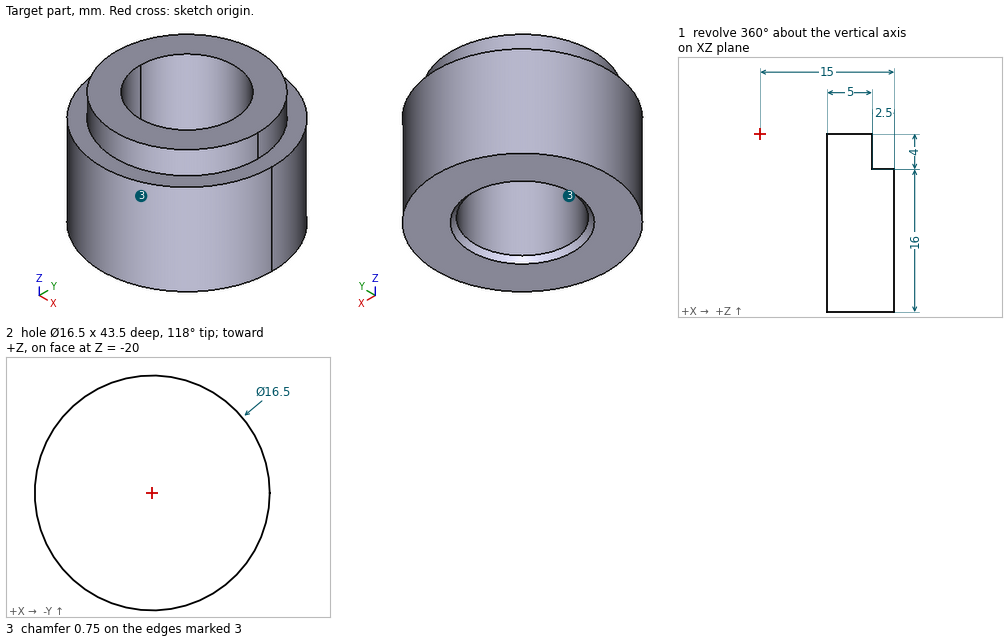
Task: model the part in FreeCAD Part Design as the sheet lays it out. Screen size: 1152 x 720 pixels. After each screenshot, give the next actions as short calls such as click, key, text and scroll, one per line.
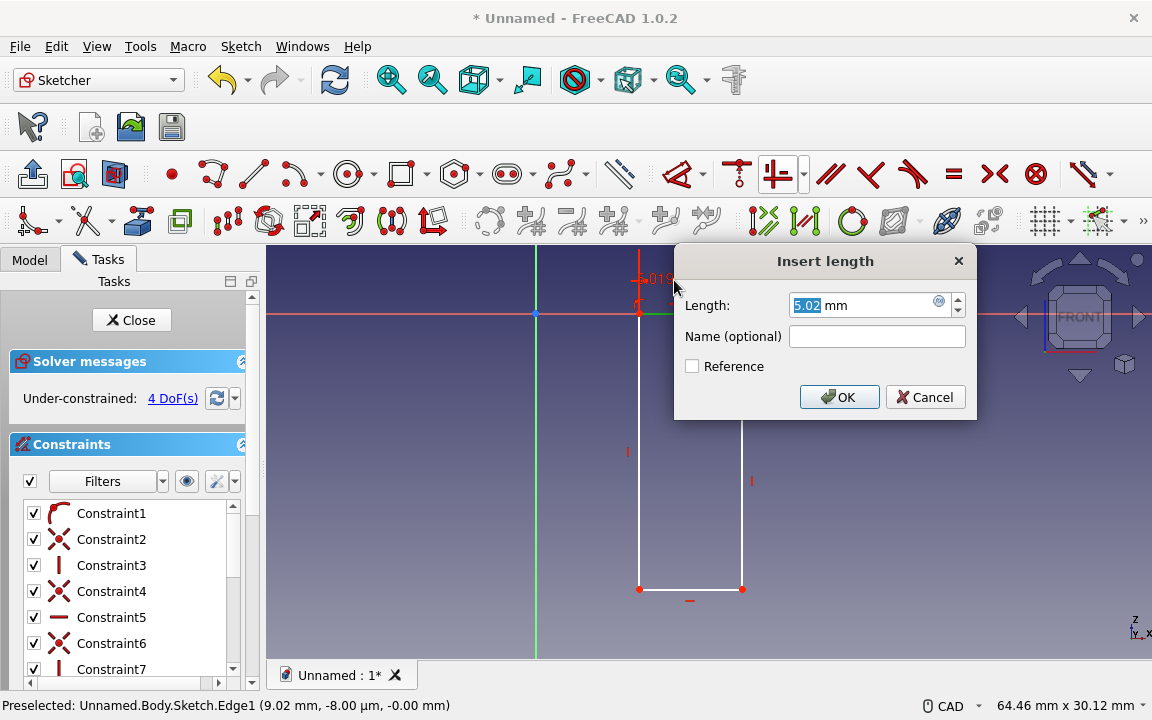
text(5)
key(Return)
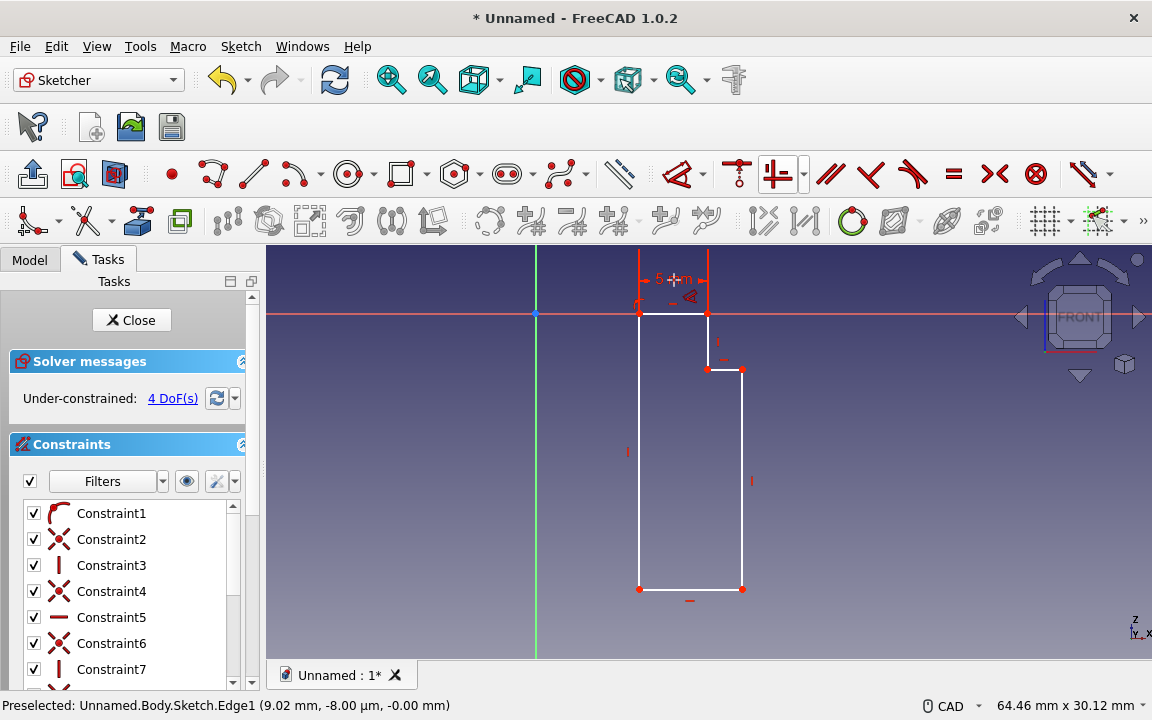
click(708, 331)
click(742, 342)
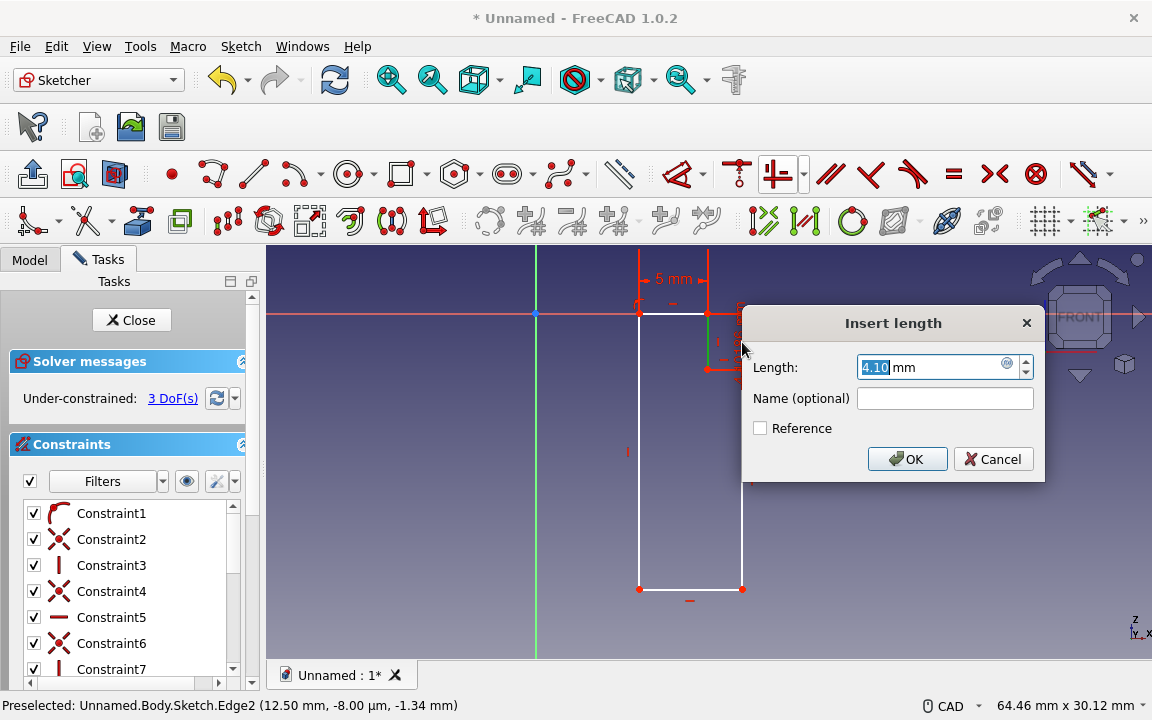
text(4)
key(Return)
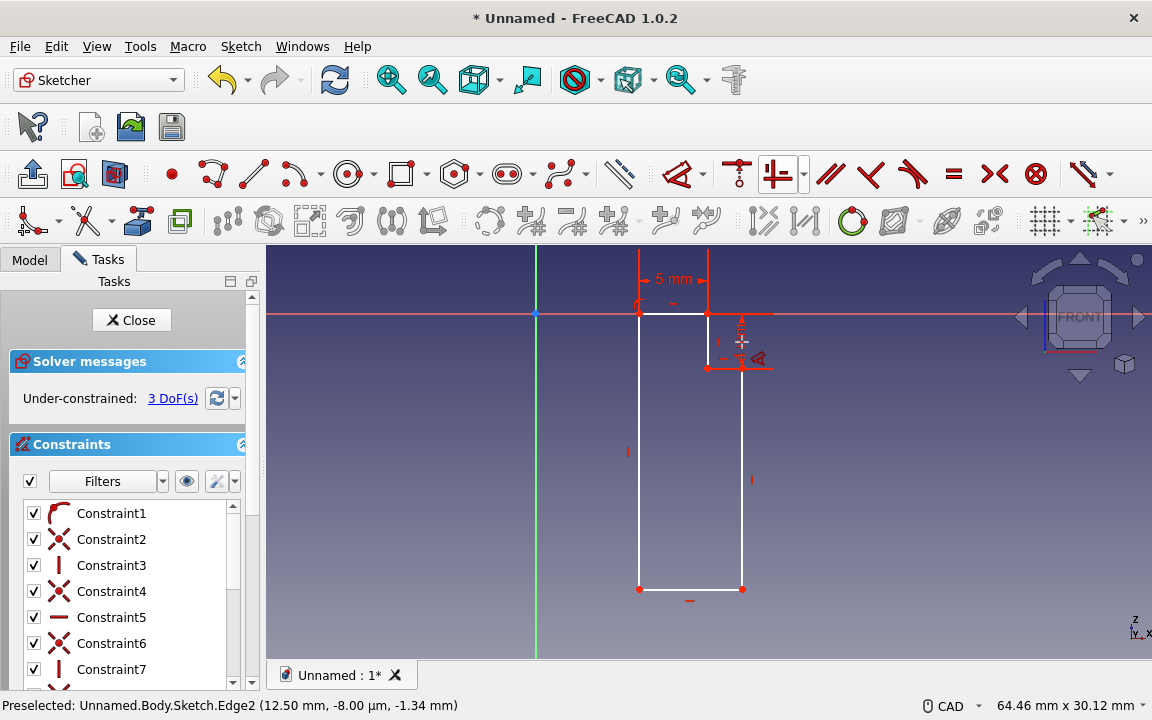
click(742, 435)
click(776, 479)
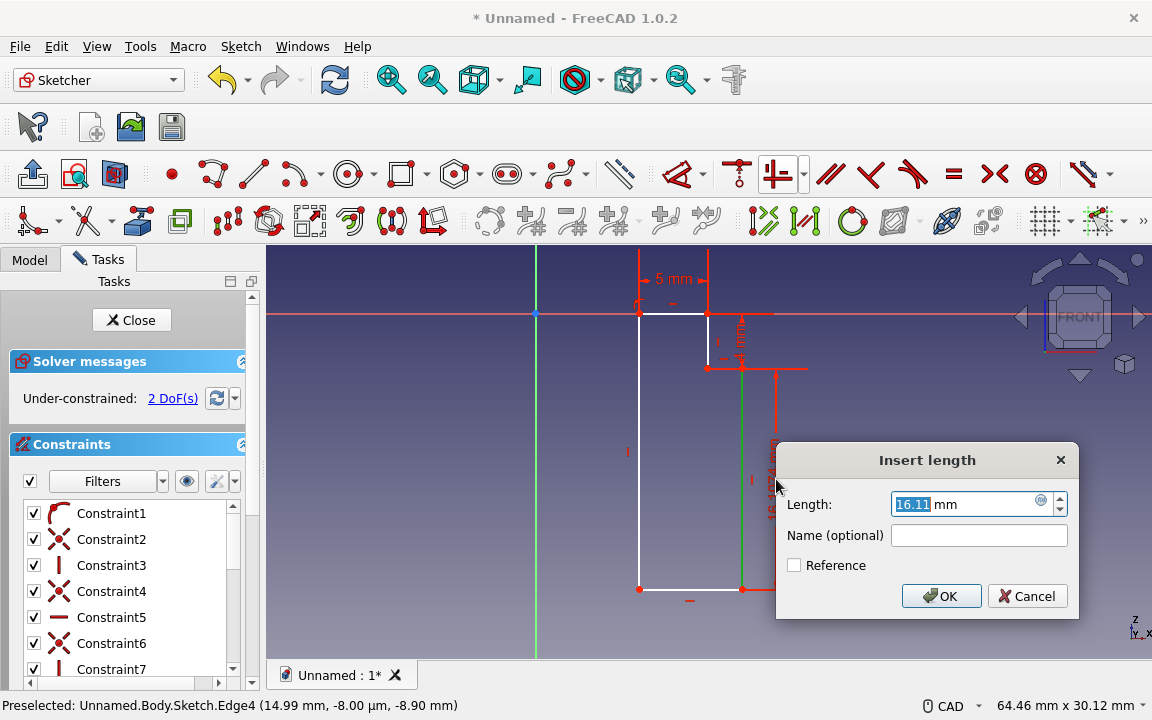
text(16)
key(Return)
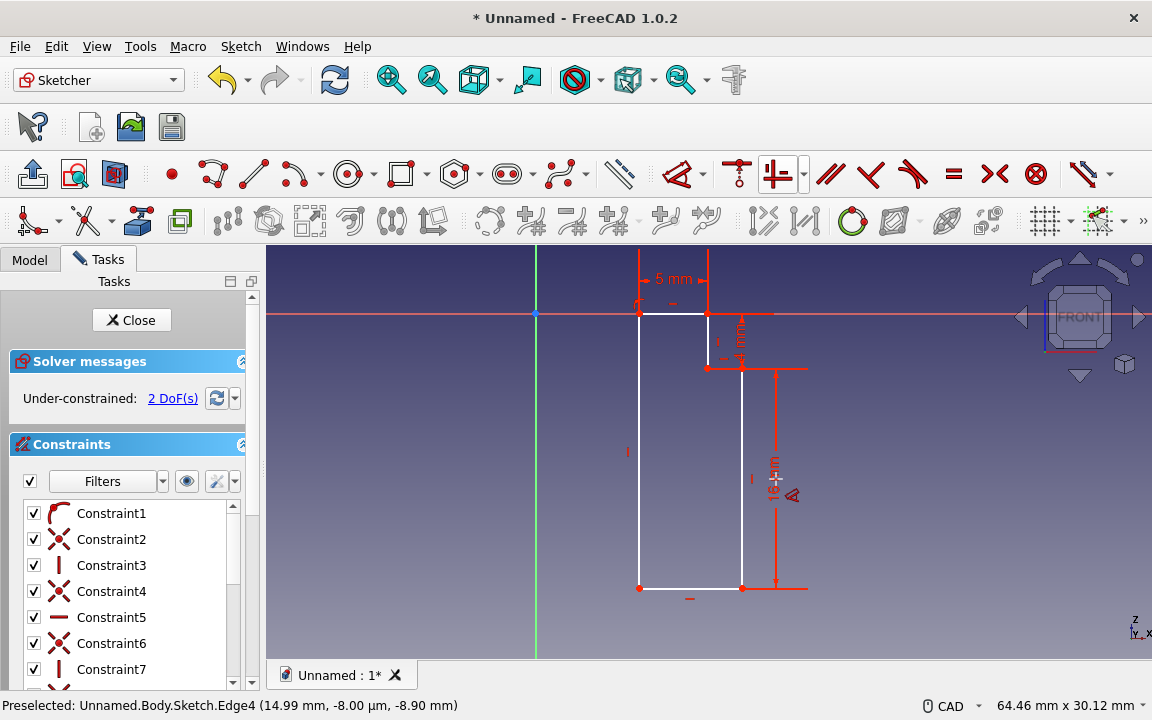
scroll(718, 369, up, 2)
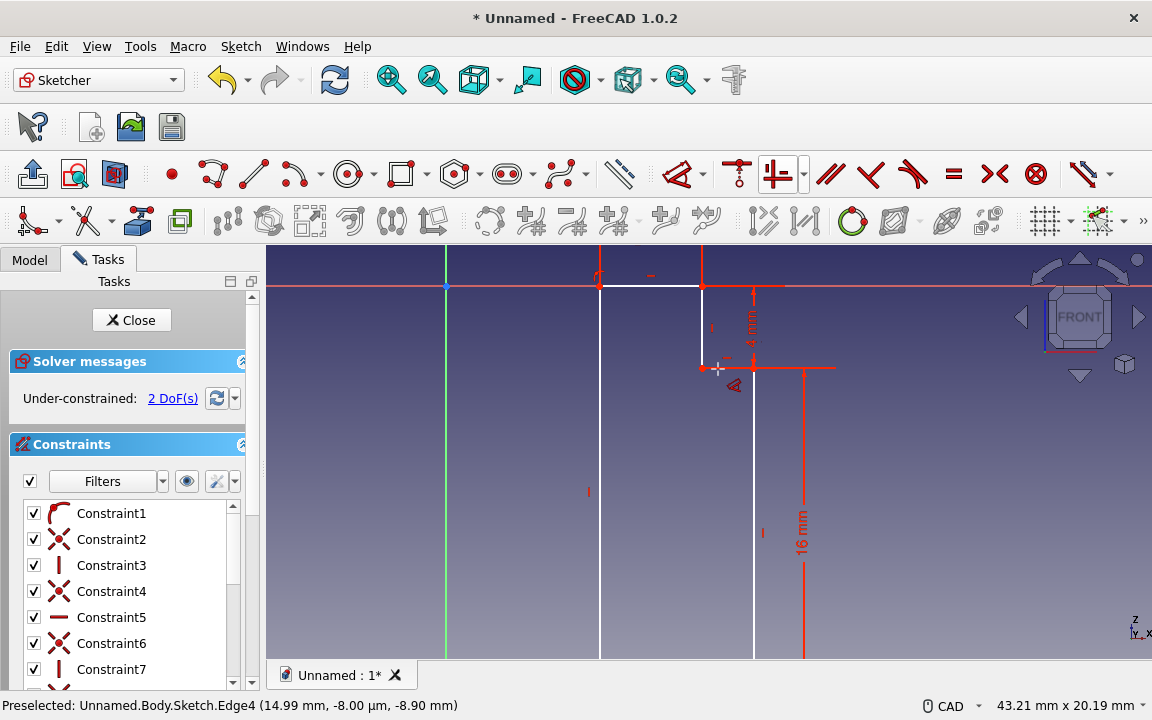
click(718, 368)
click(728, 402)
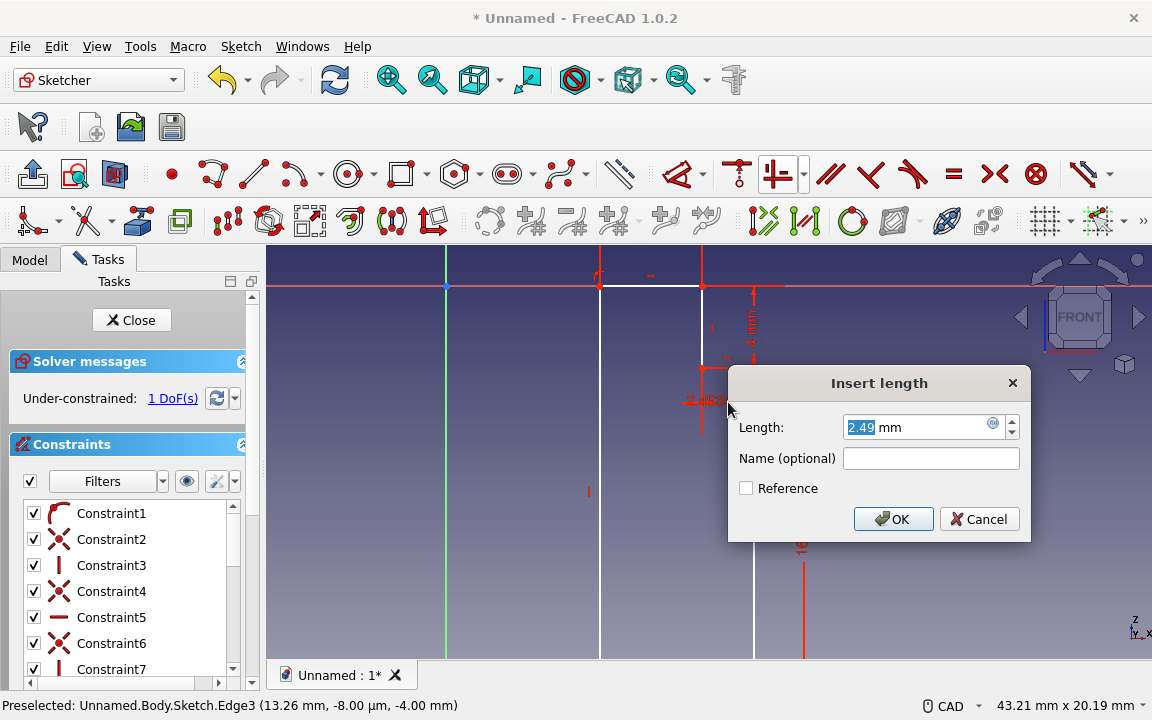
text(2.5)
key(Return)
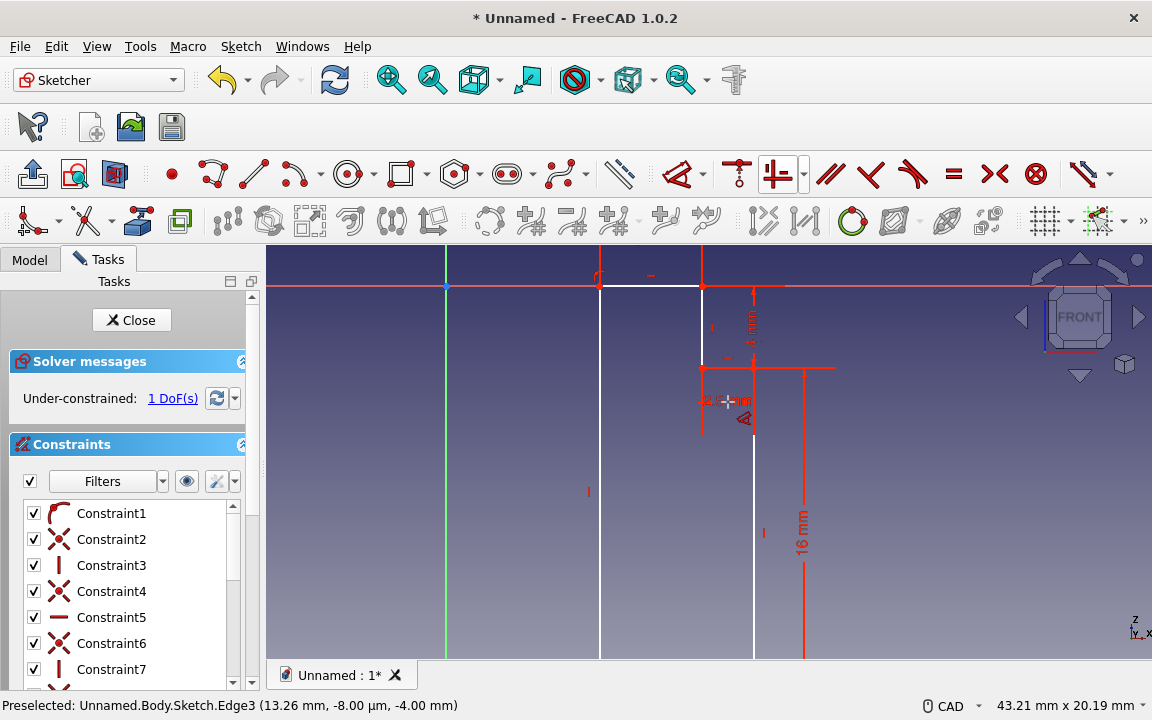
click(754, 368)
click(529, 402)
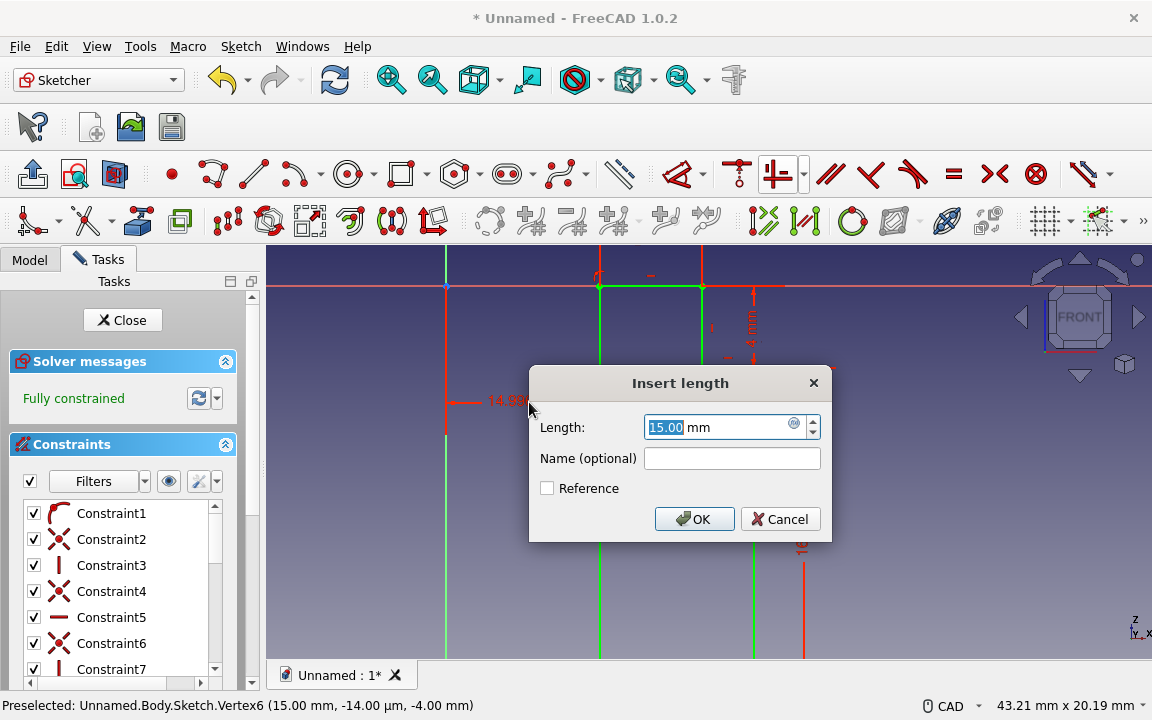
text(15)
key(Return)
key(Escape)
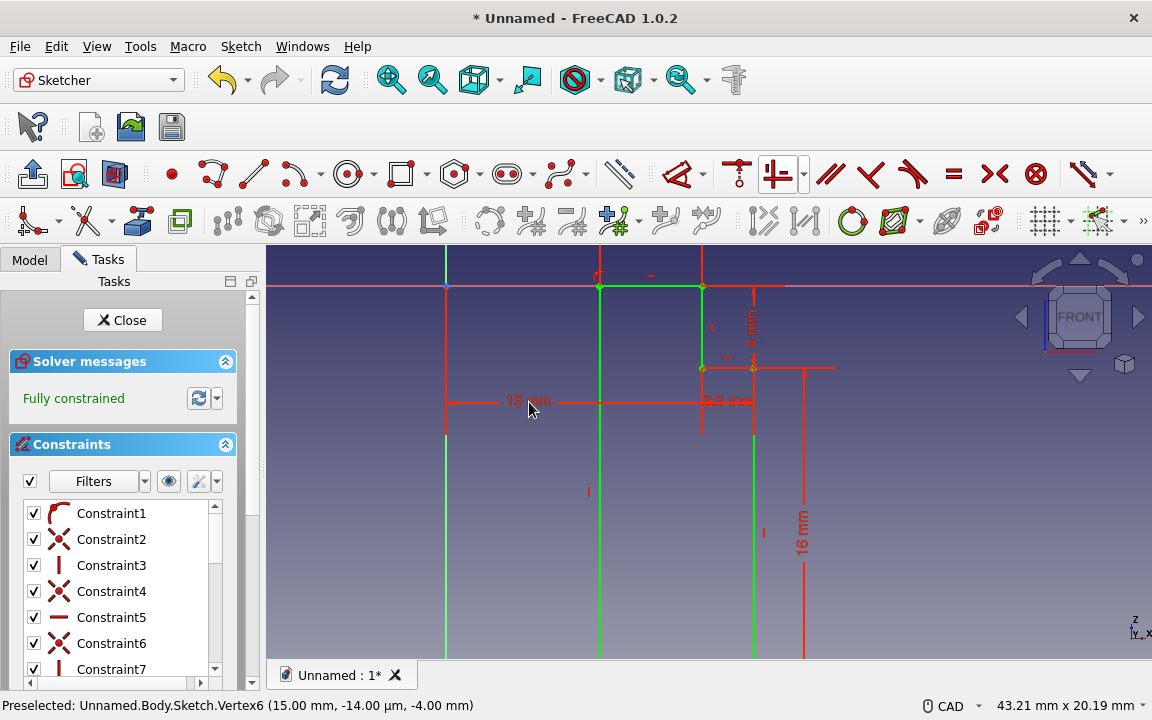
click(123, 320)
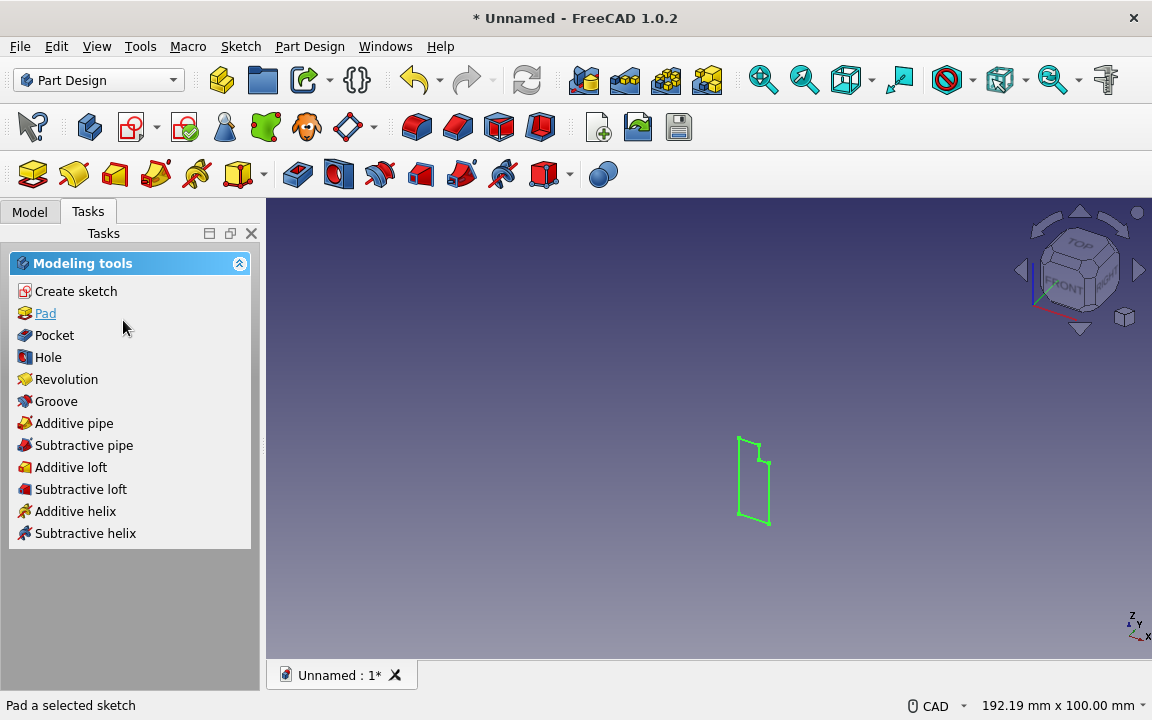
click(74, 174)